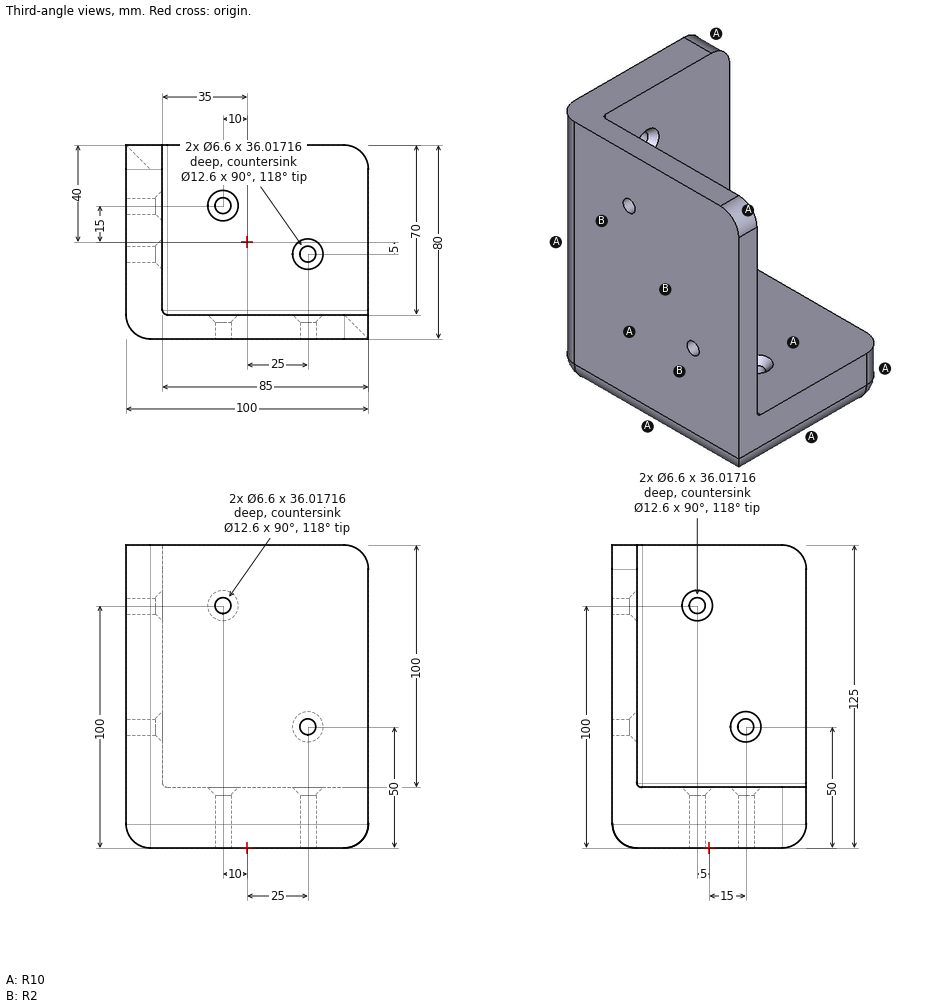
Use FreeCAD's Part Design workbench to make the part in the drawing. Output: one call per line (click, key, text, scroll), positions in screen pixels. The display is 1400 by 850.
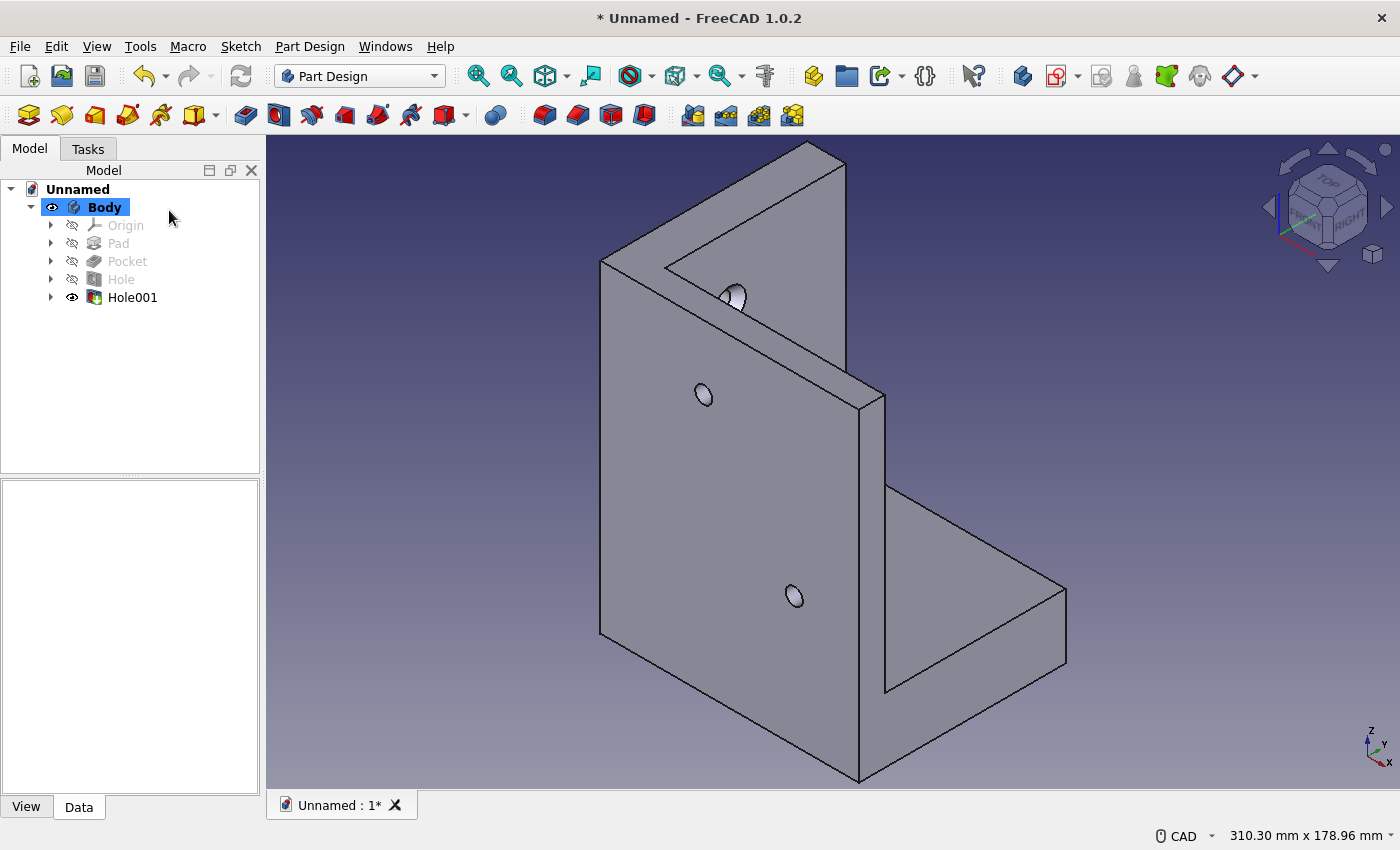
click(897, 595)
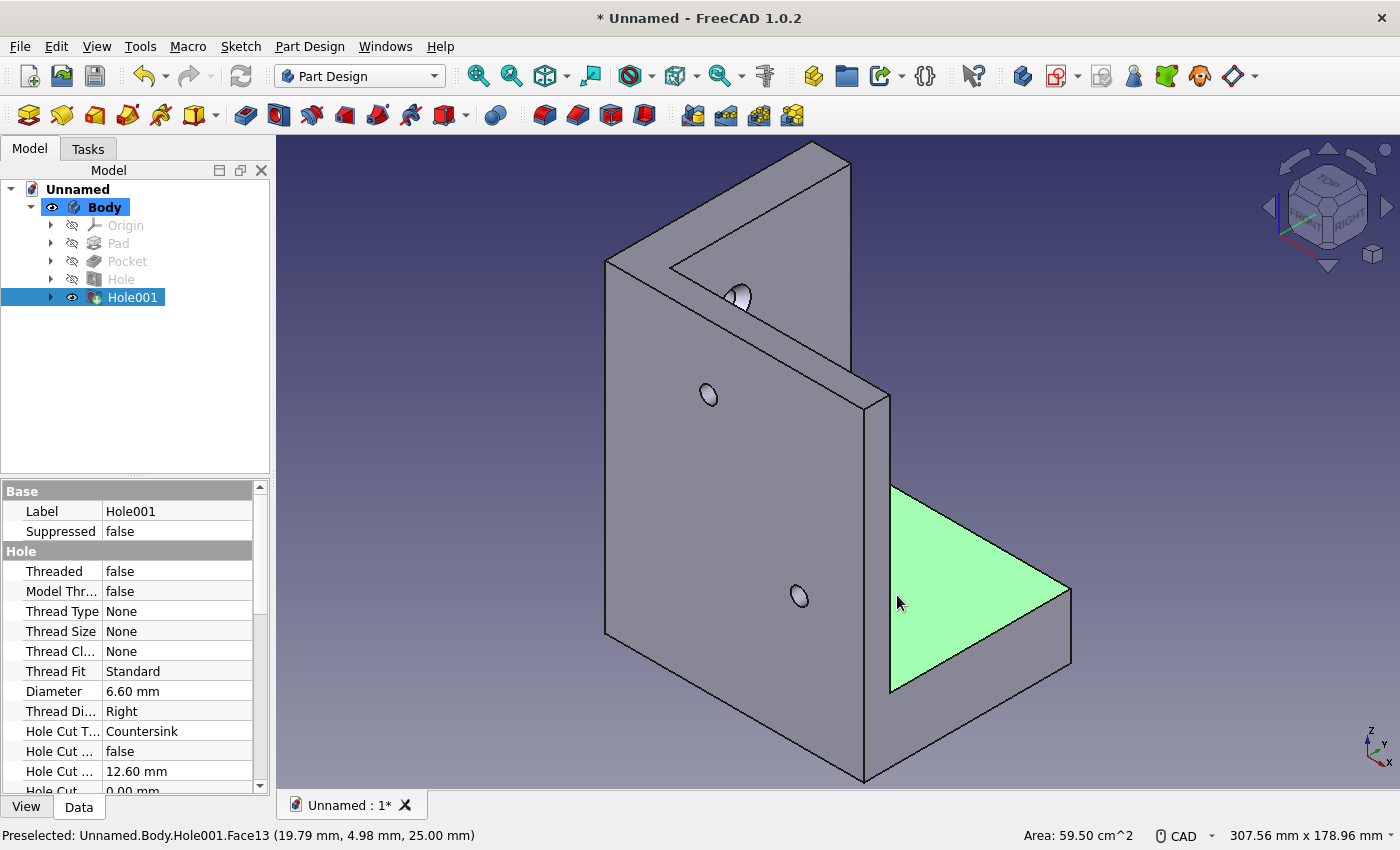
click(1056, 76)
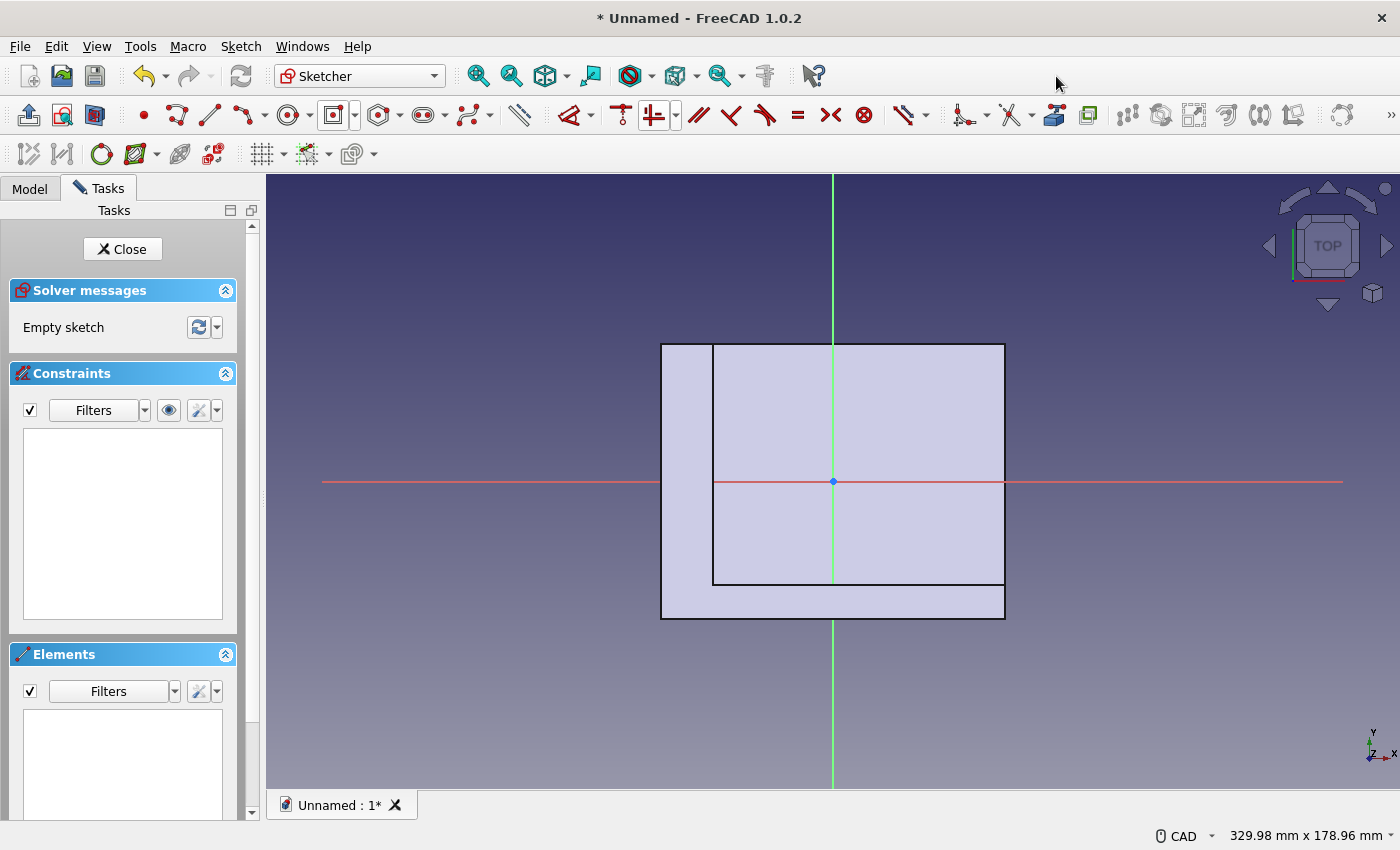
key(q)
key(s)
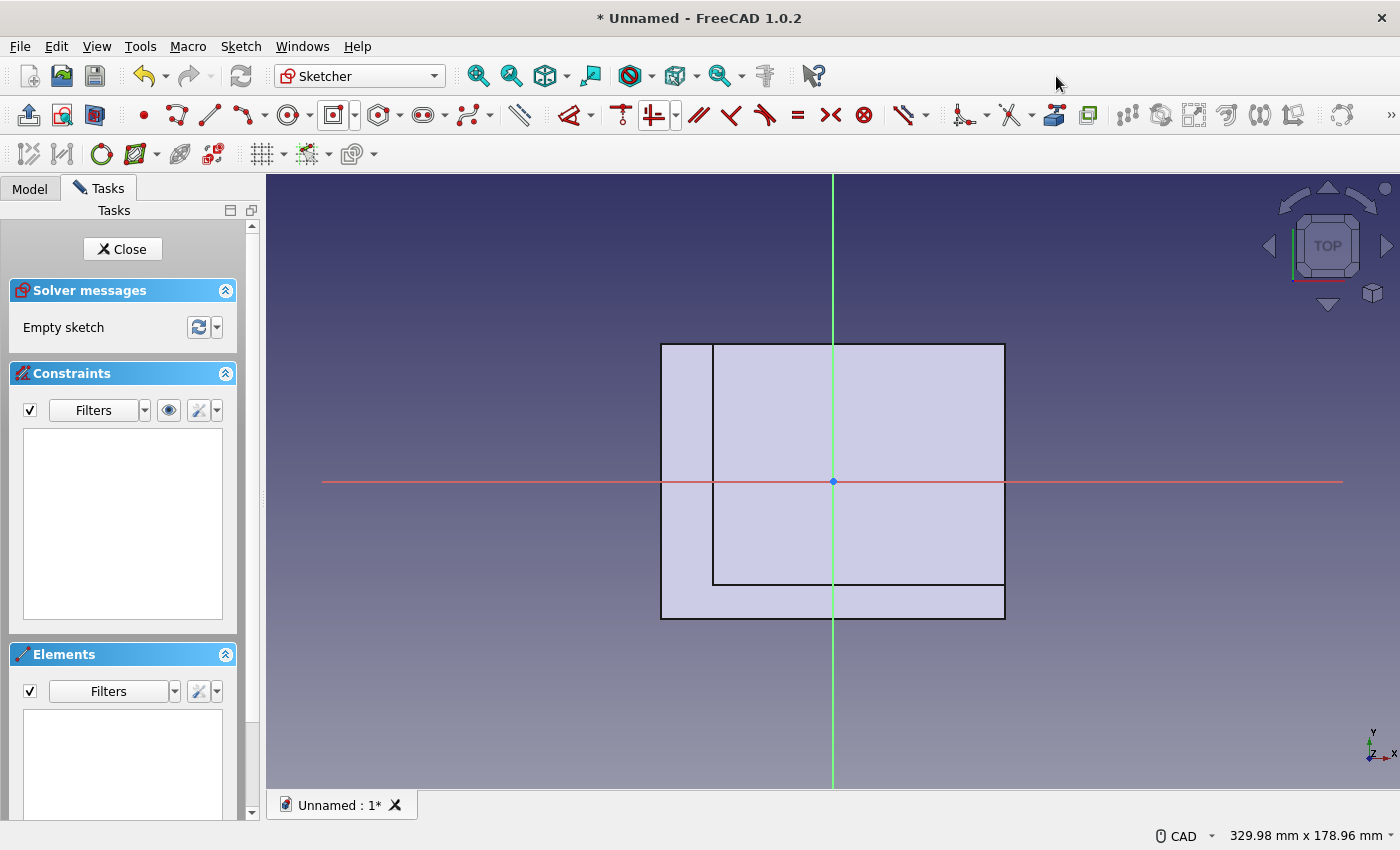
scroll(890, 459, up, 7)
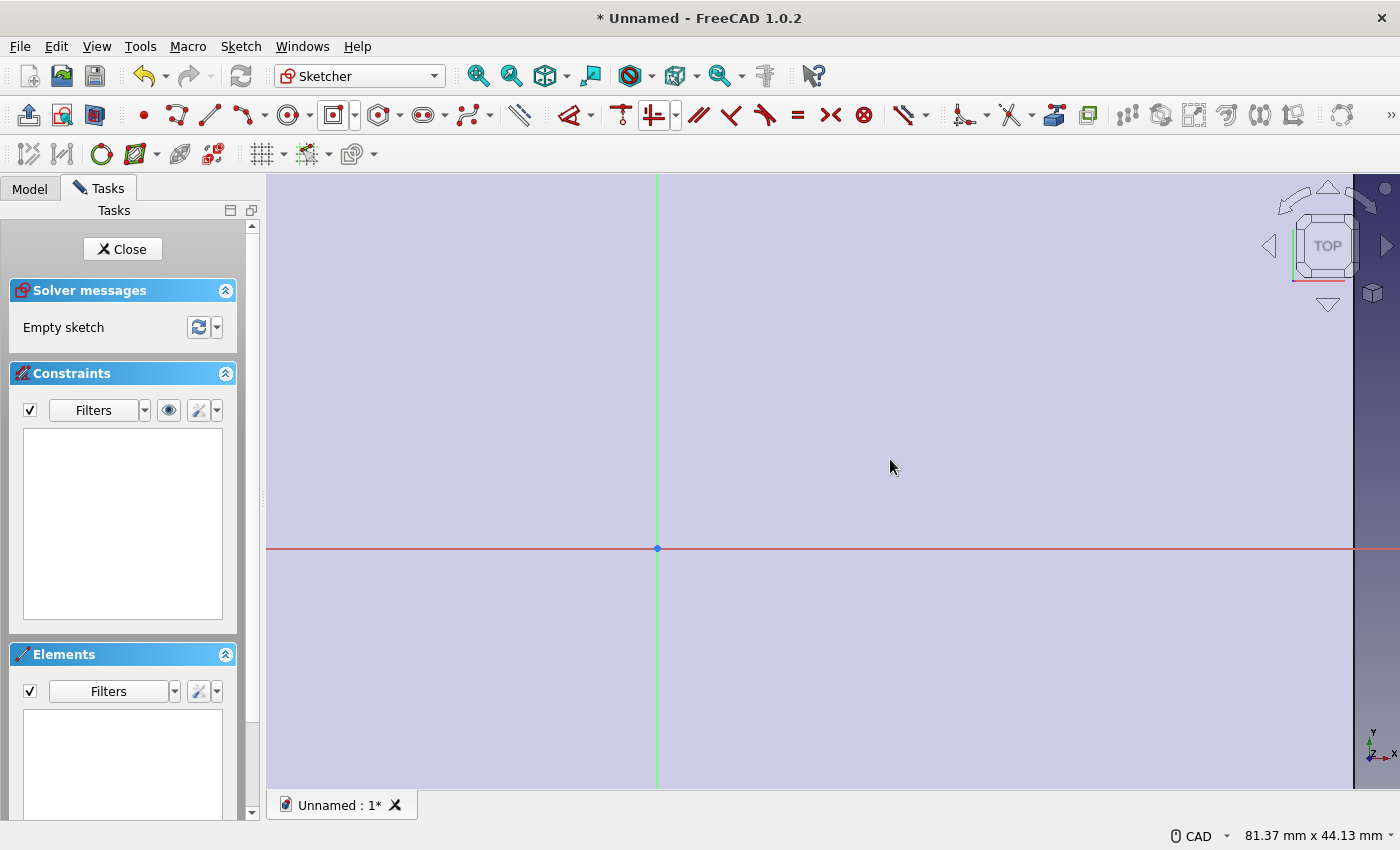
click(288, 116)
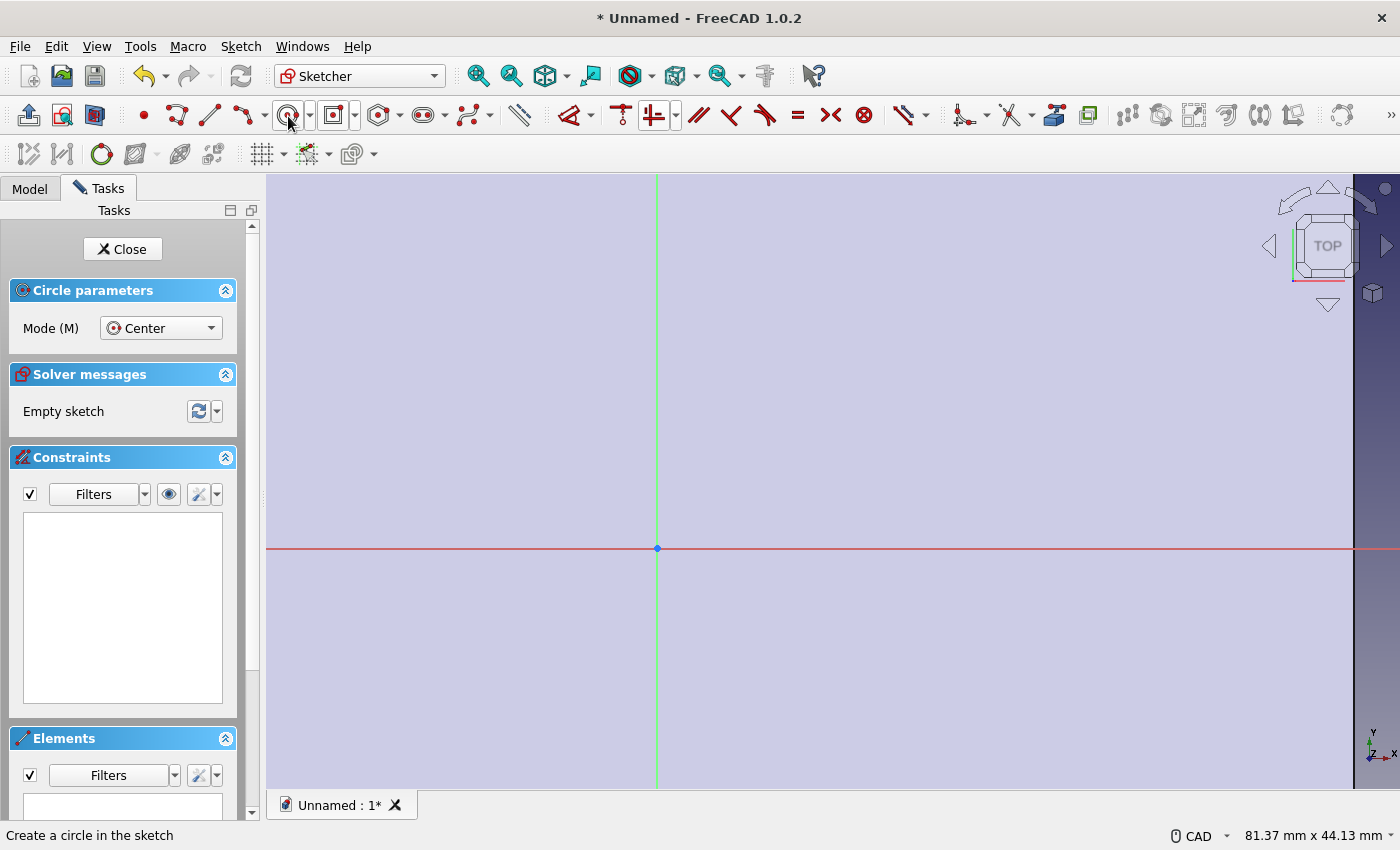
click(1006, 619)
move(1038, 586)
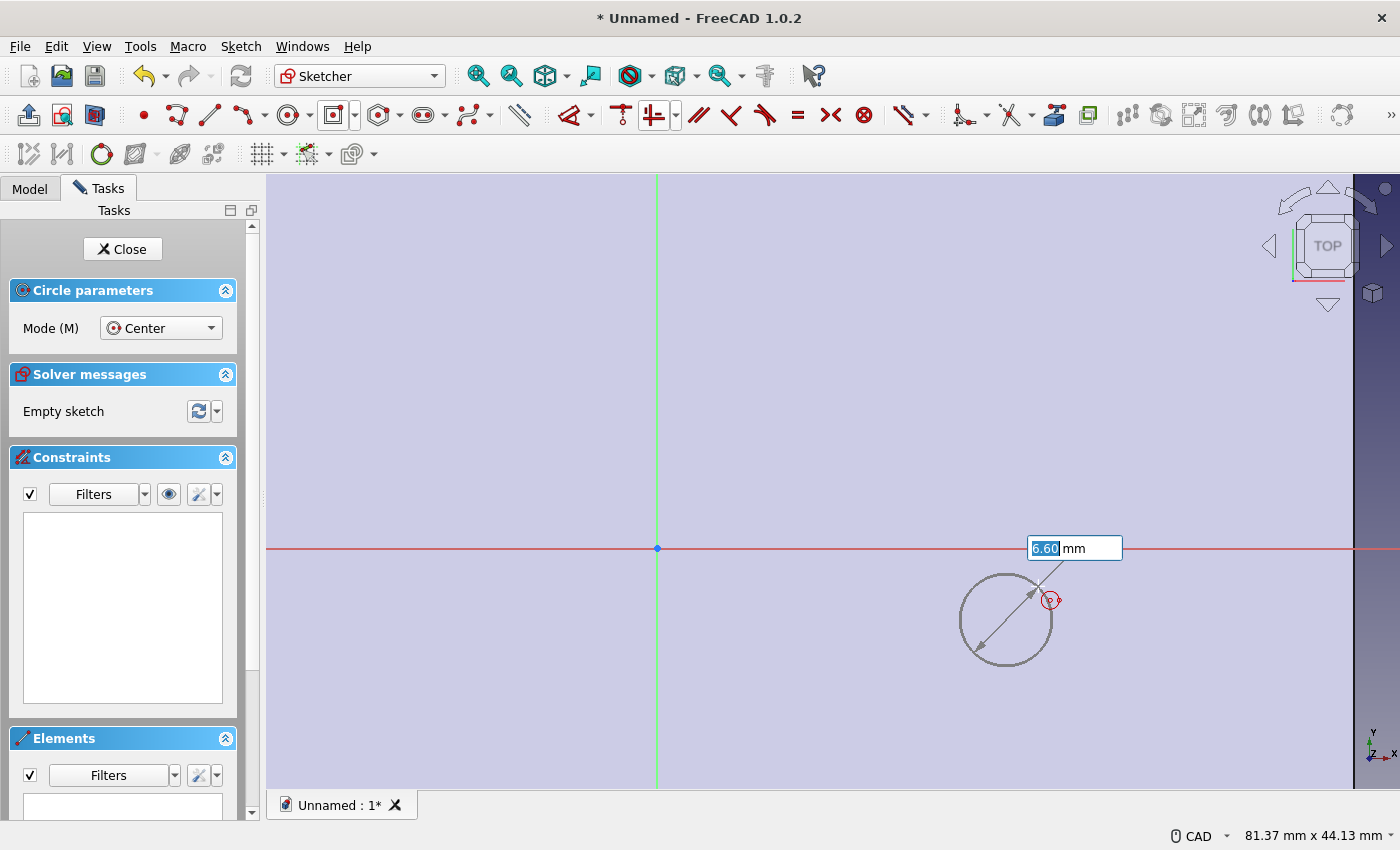
text(6.6)
key(Return)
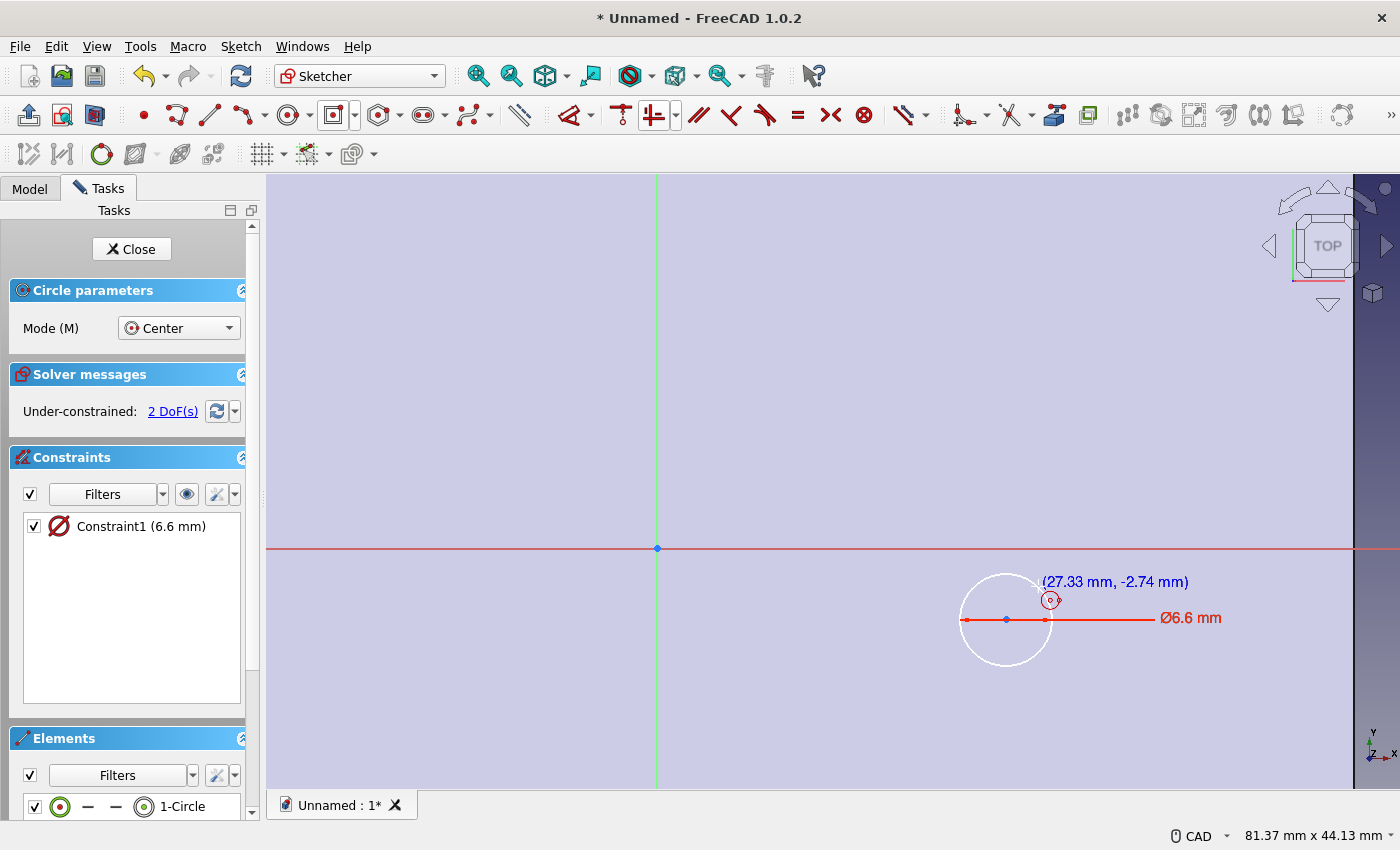
click(518, 340)
move(550, 307)